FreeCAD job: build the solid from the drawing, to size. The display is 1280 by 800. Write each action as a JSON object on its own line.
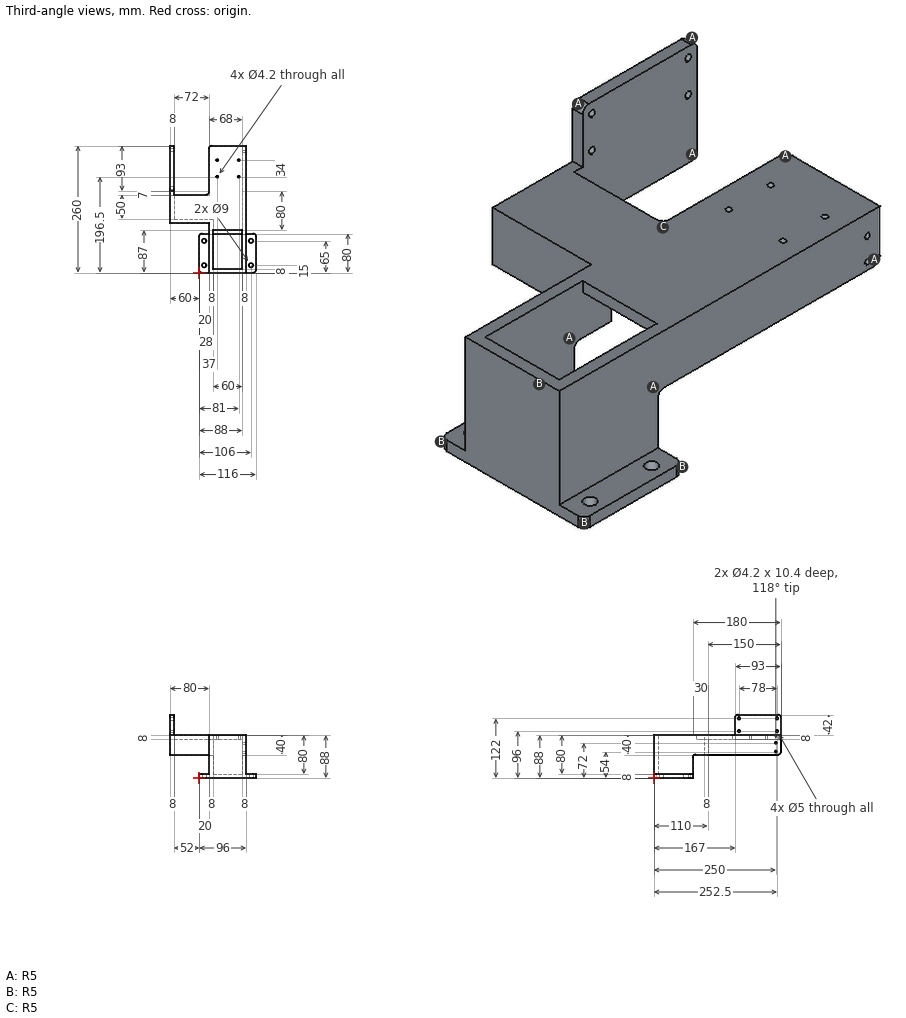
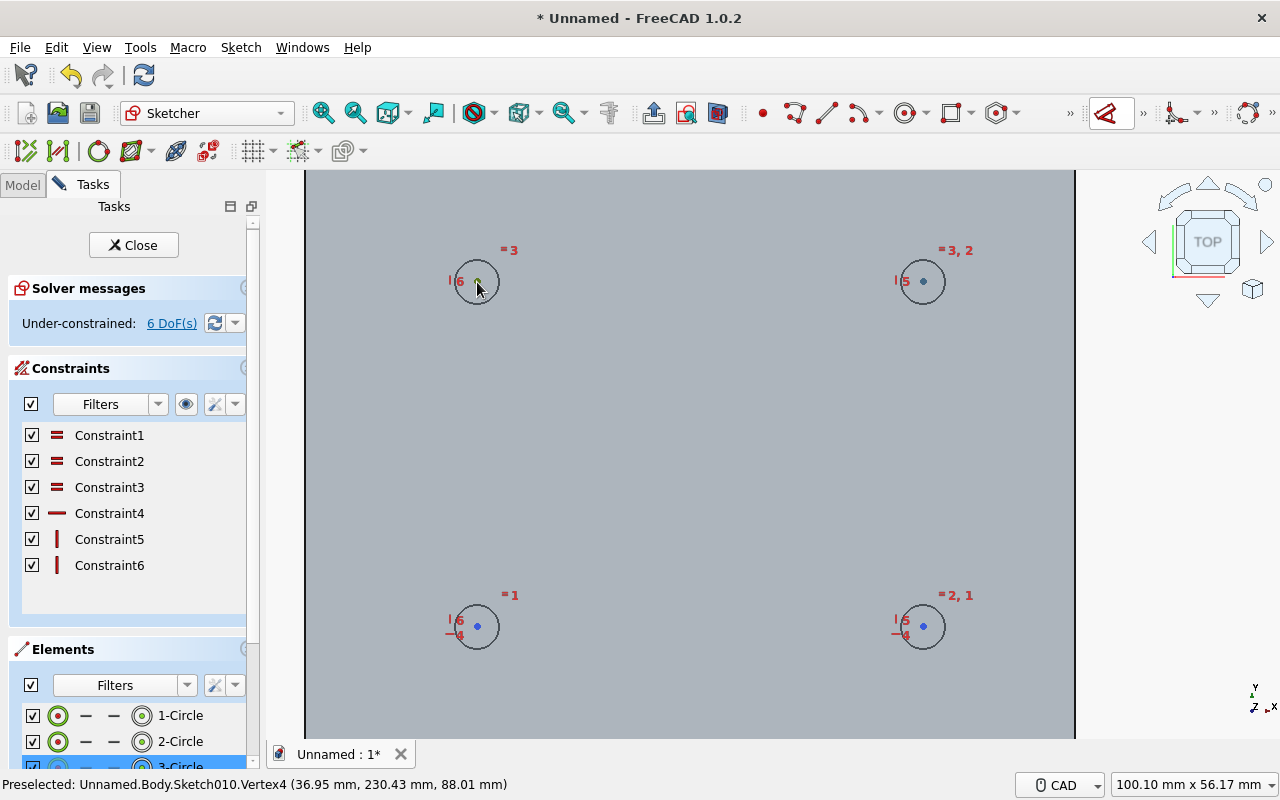
{"action": "key", "text": "h"}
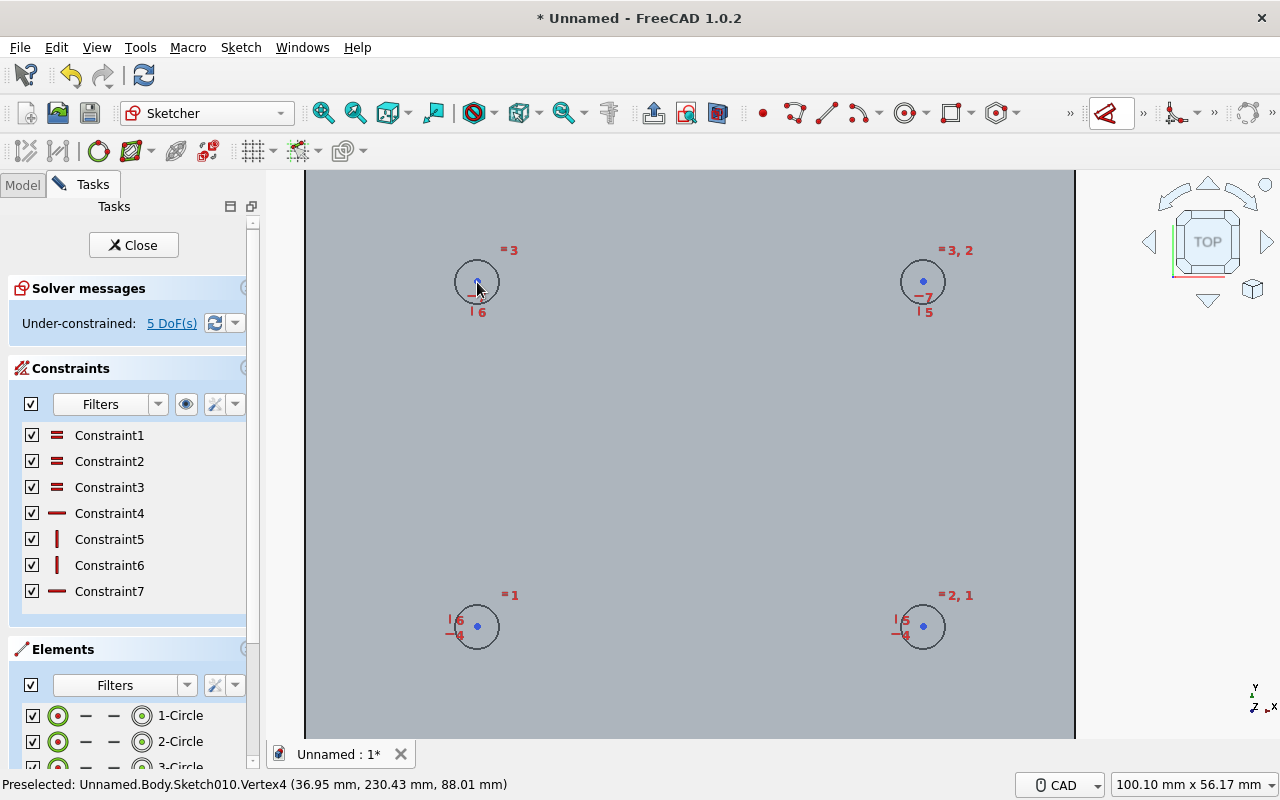
{"action": "left_click", "coordinate": [492, 611]}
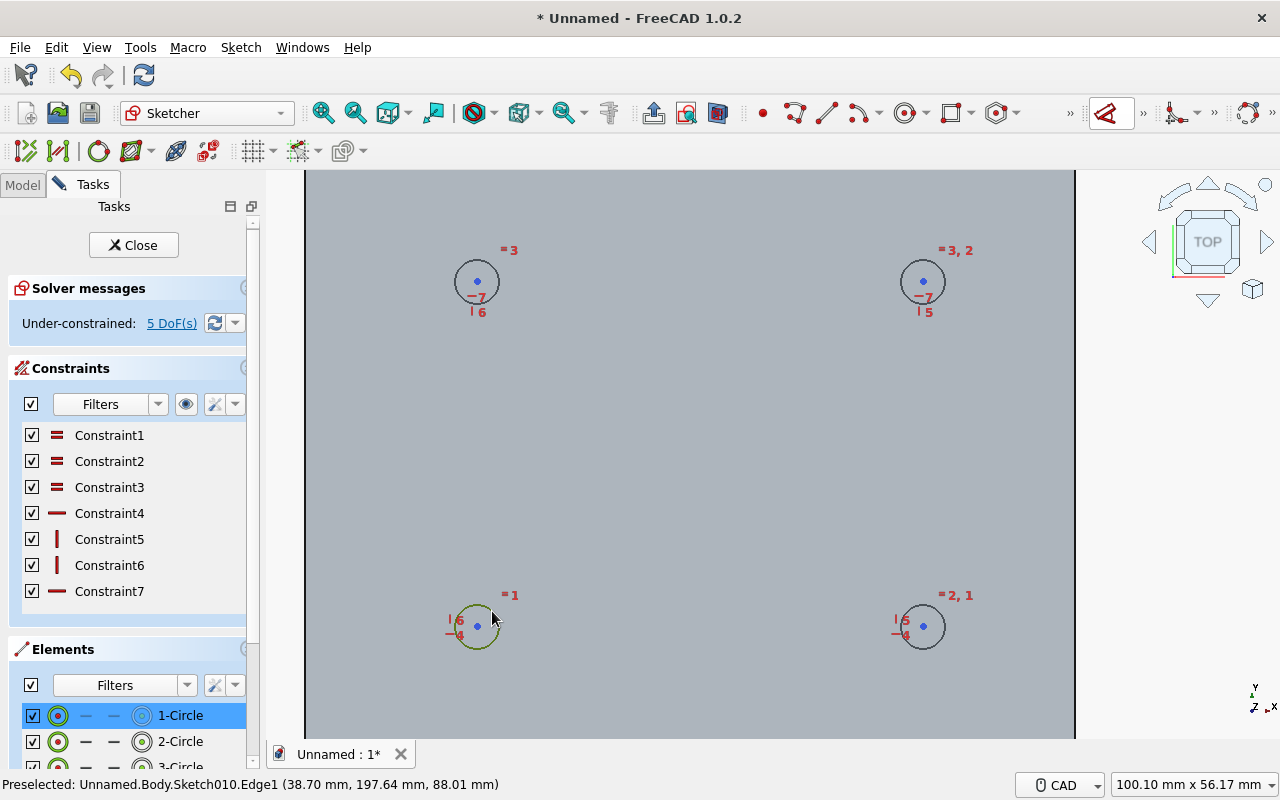
{"action": "left_click", "coordinate": [1128, 114]}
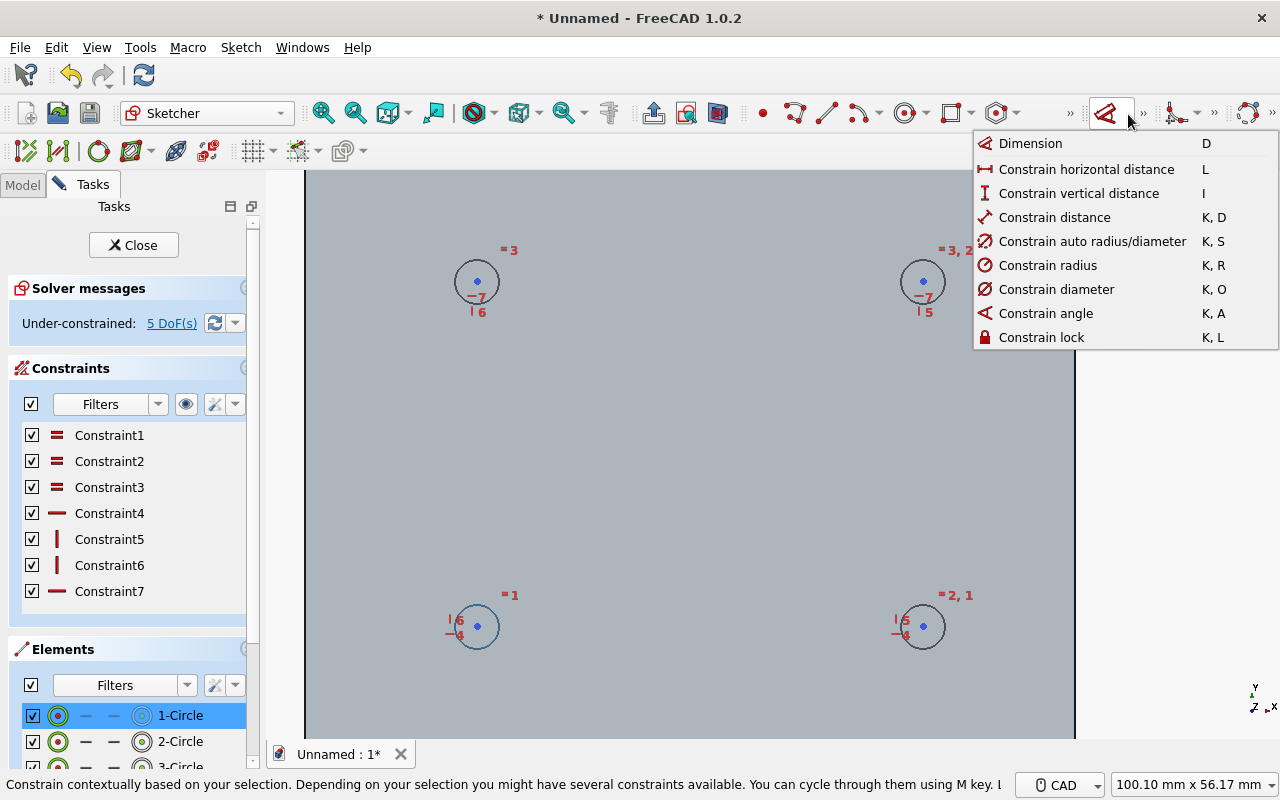
{"action": "left_click", "coordinate": [1126, 289]}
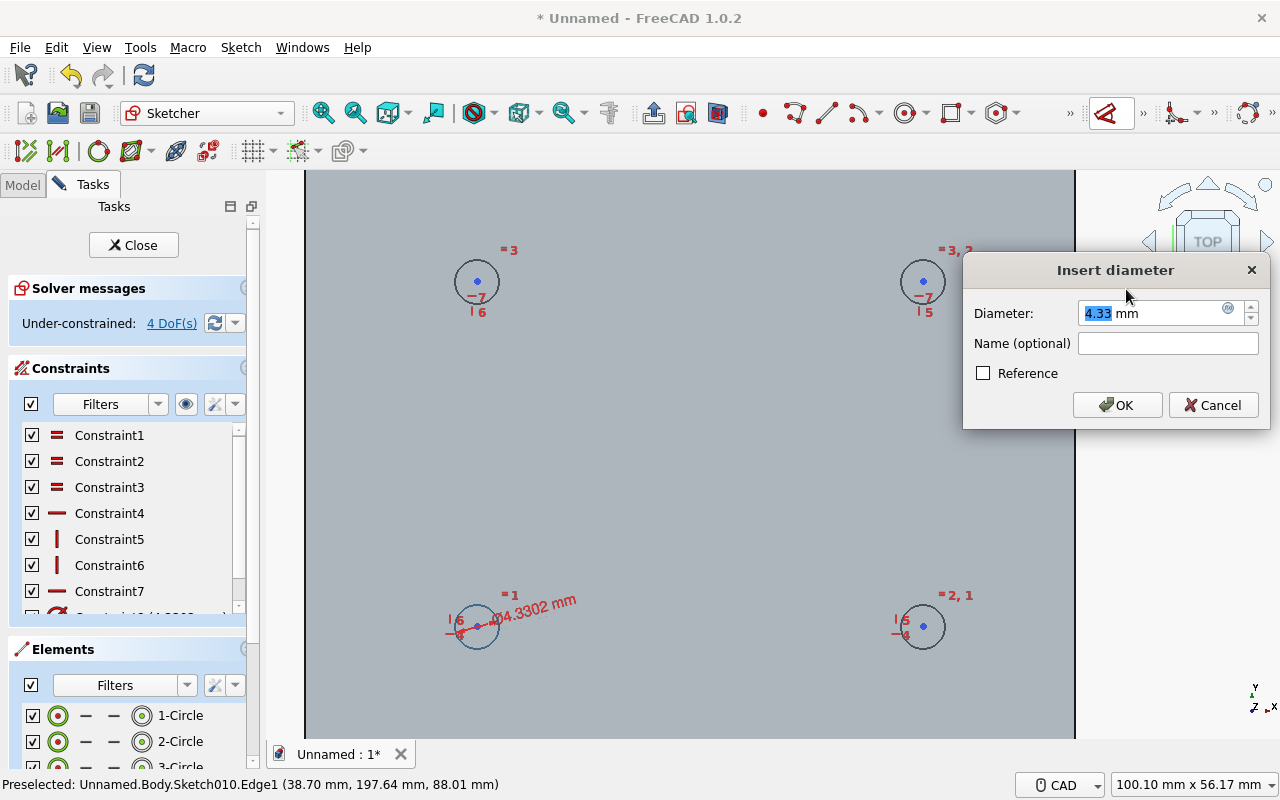
{"action": "type", "text": "4.2"}
{"action": "key", "text": "Return"}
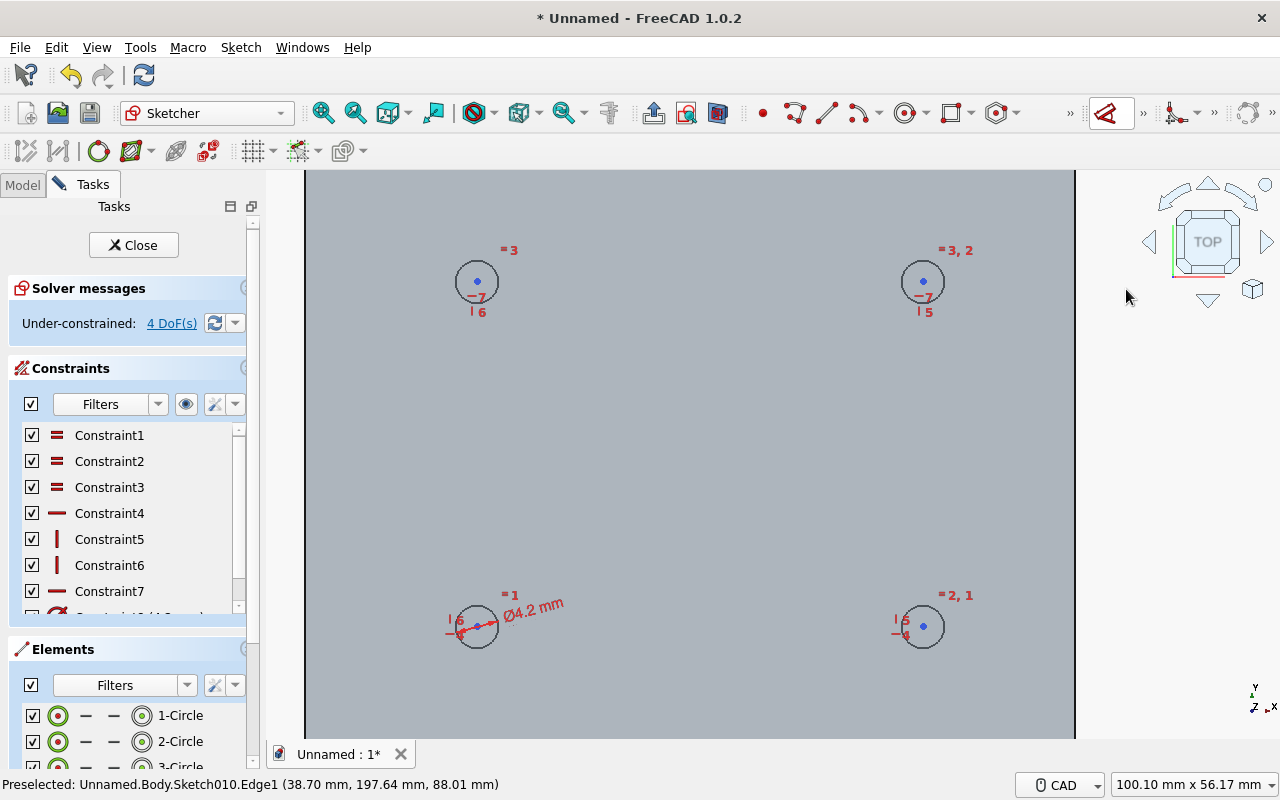
{"action": "left_click", "coordinate": [477, 627]}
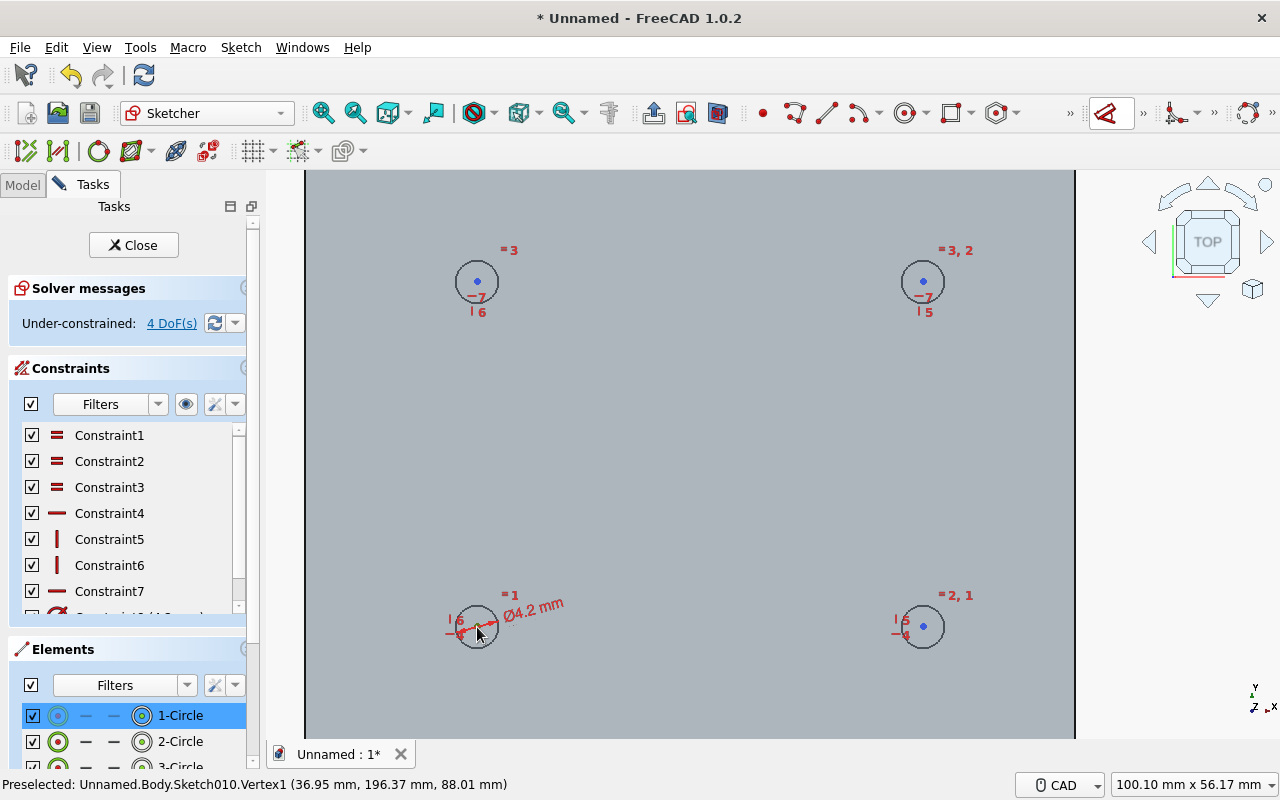
{"action": "key", "text": "l"}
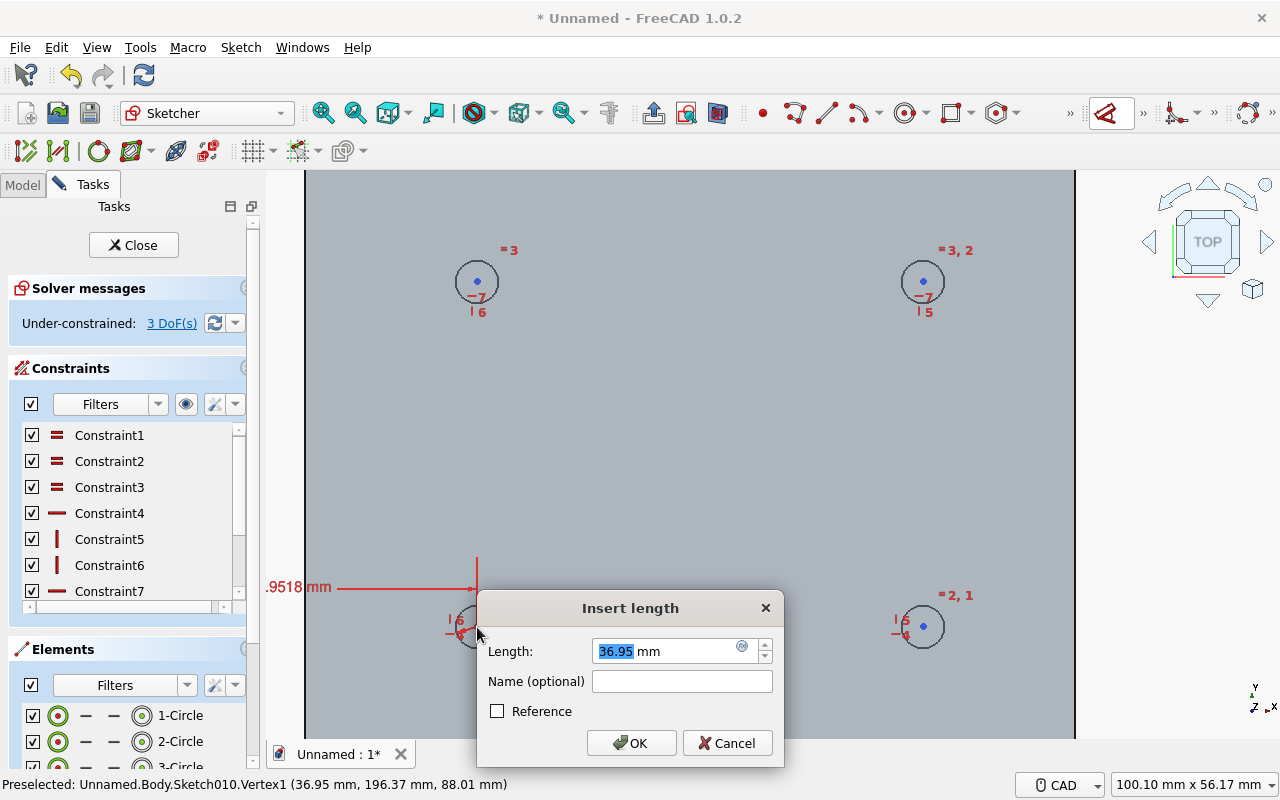
{"action": "type", "text": "37"}
{"action": "key", "text": "Return"}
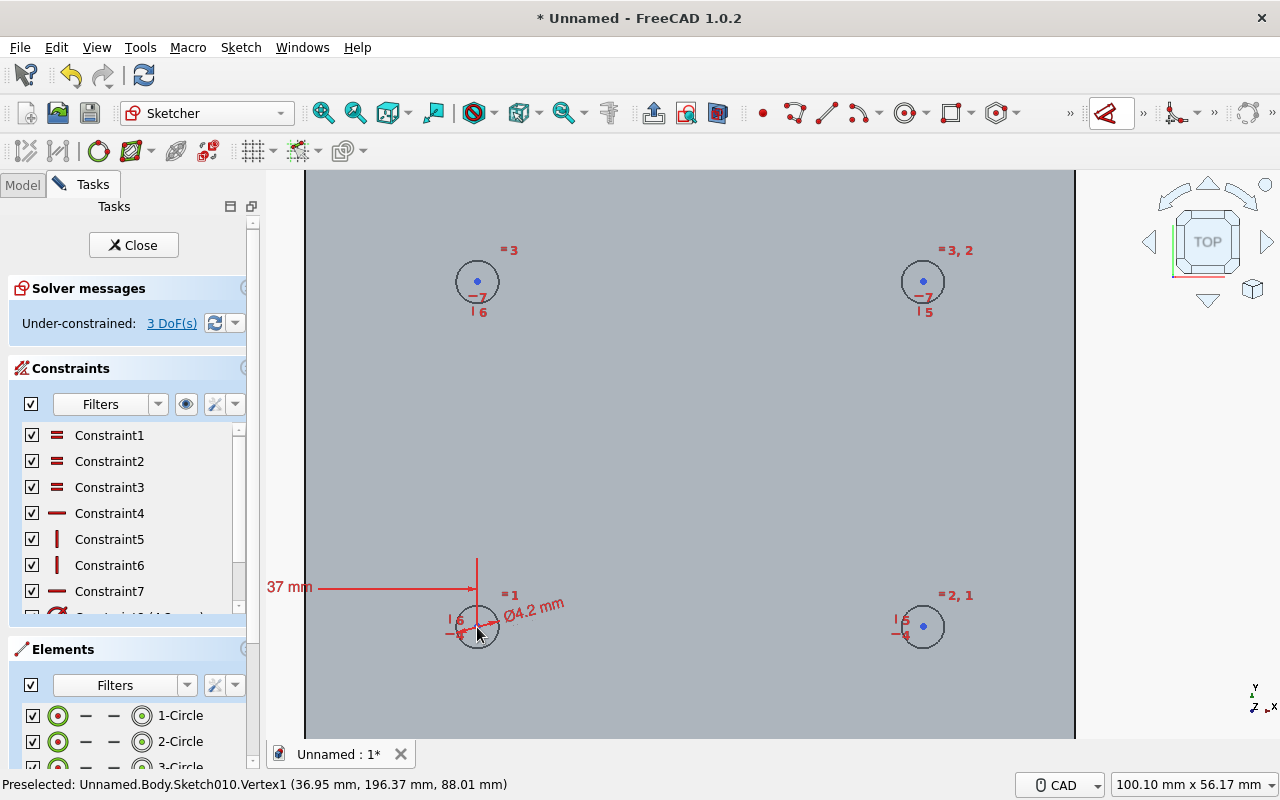
{"action": "left_click", "coordinate": [923, 627]}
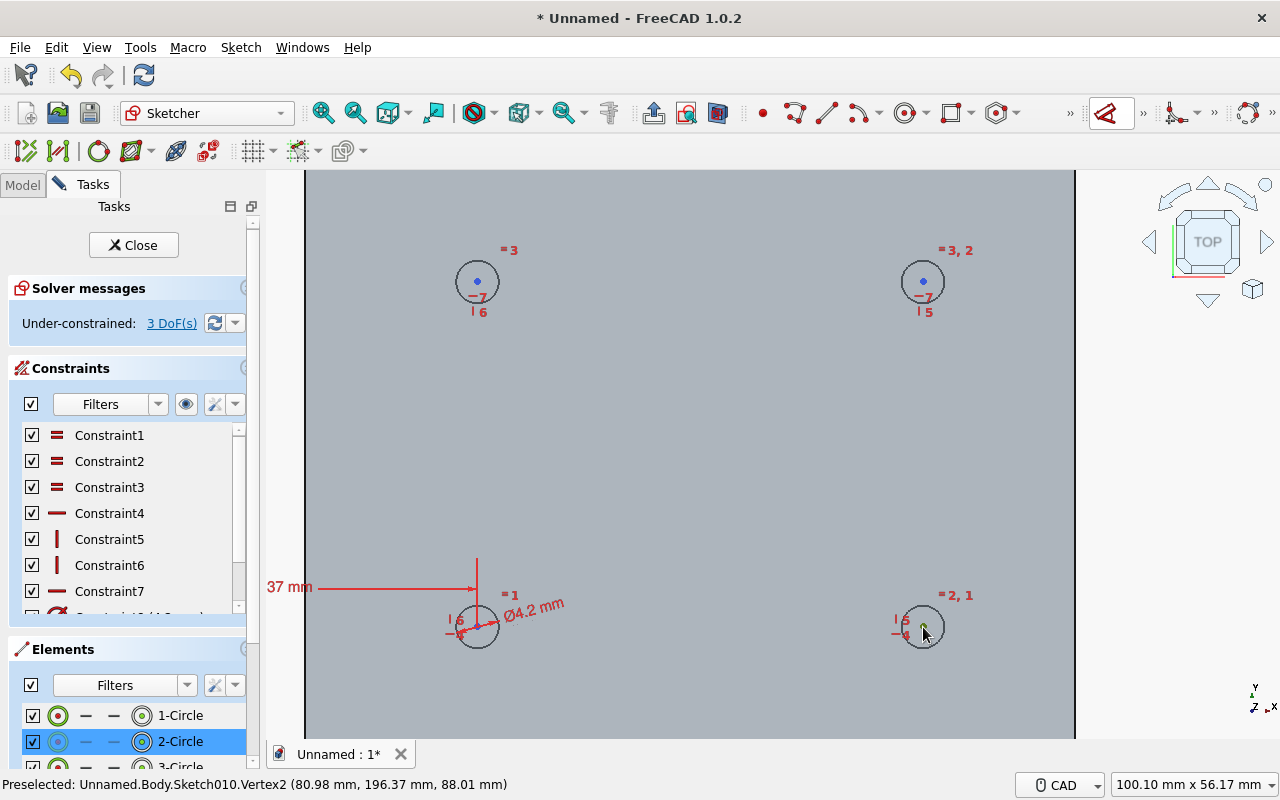
{"action": "left_click", "coordinate": [1128, 114]}